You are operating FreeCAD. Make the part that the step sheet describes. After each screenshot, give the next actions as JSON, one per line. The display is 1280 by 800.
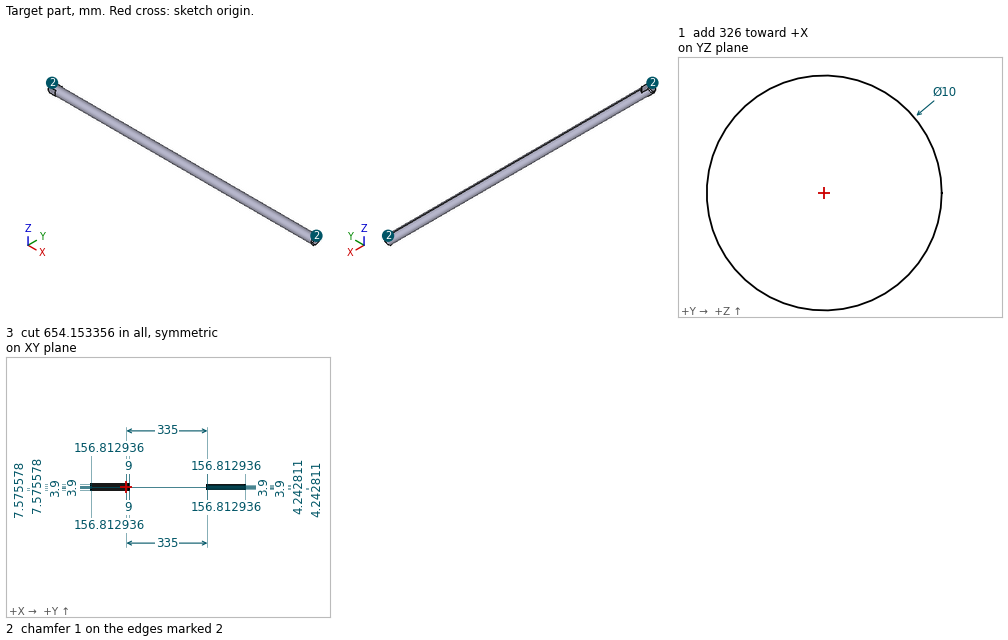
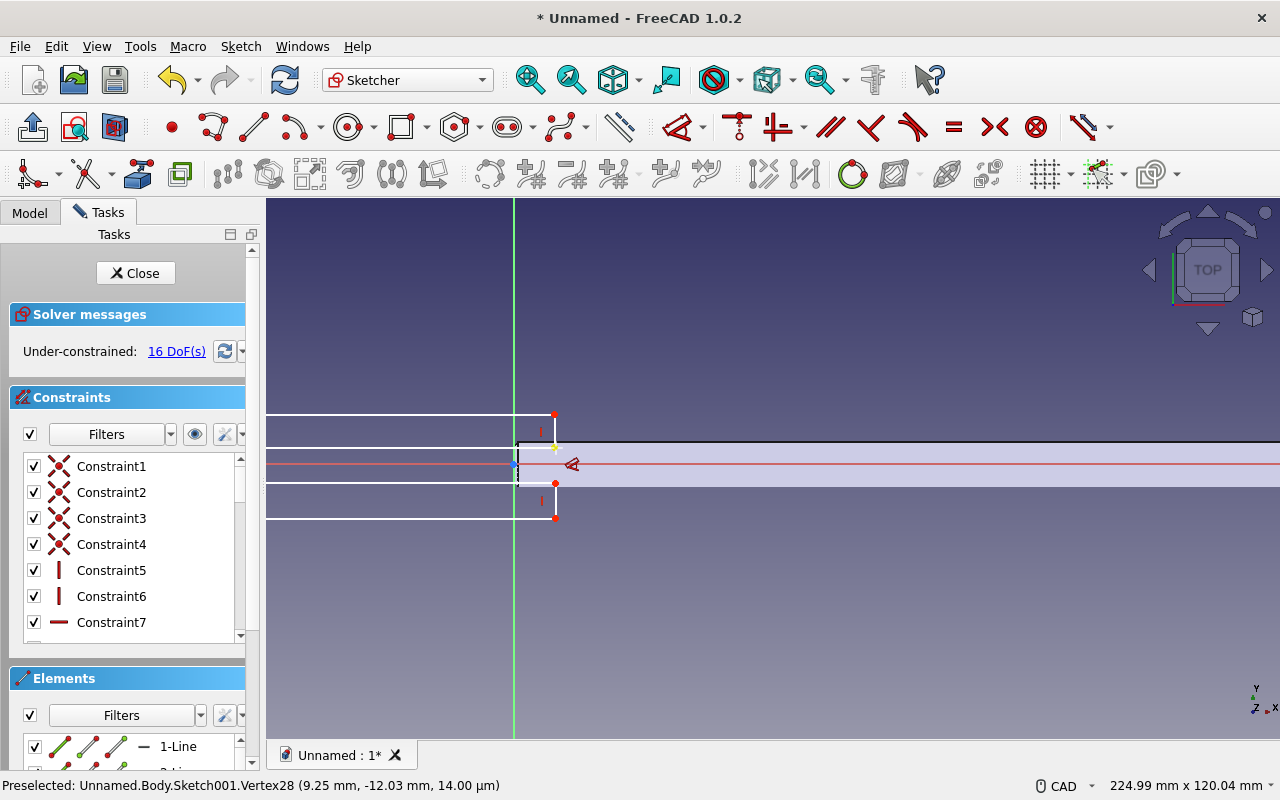
{"action": "left_click", "coordinate": [555, 448]}
{"action": "left_click", "coordinate": [534, 498]}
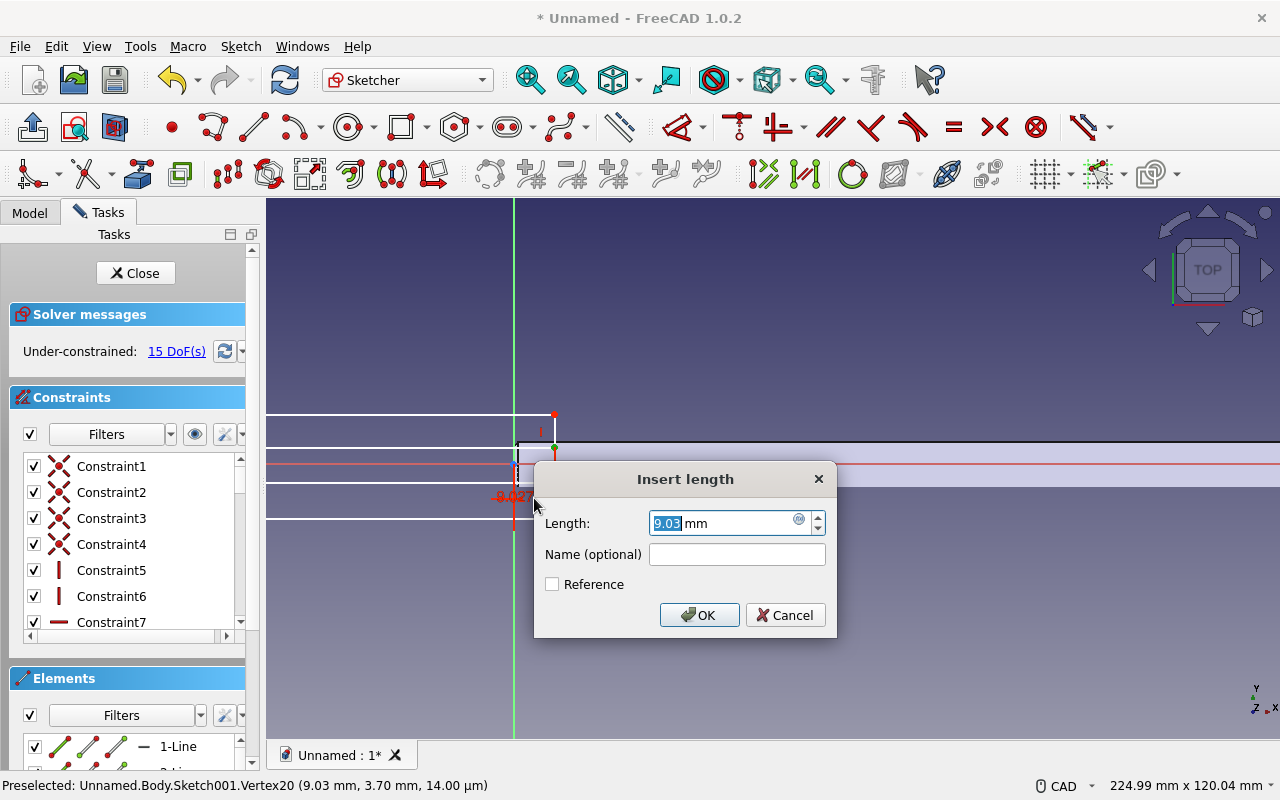
{"action": "type", "text": "9"}
{"action": "key", "text": "Return"}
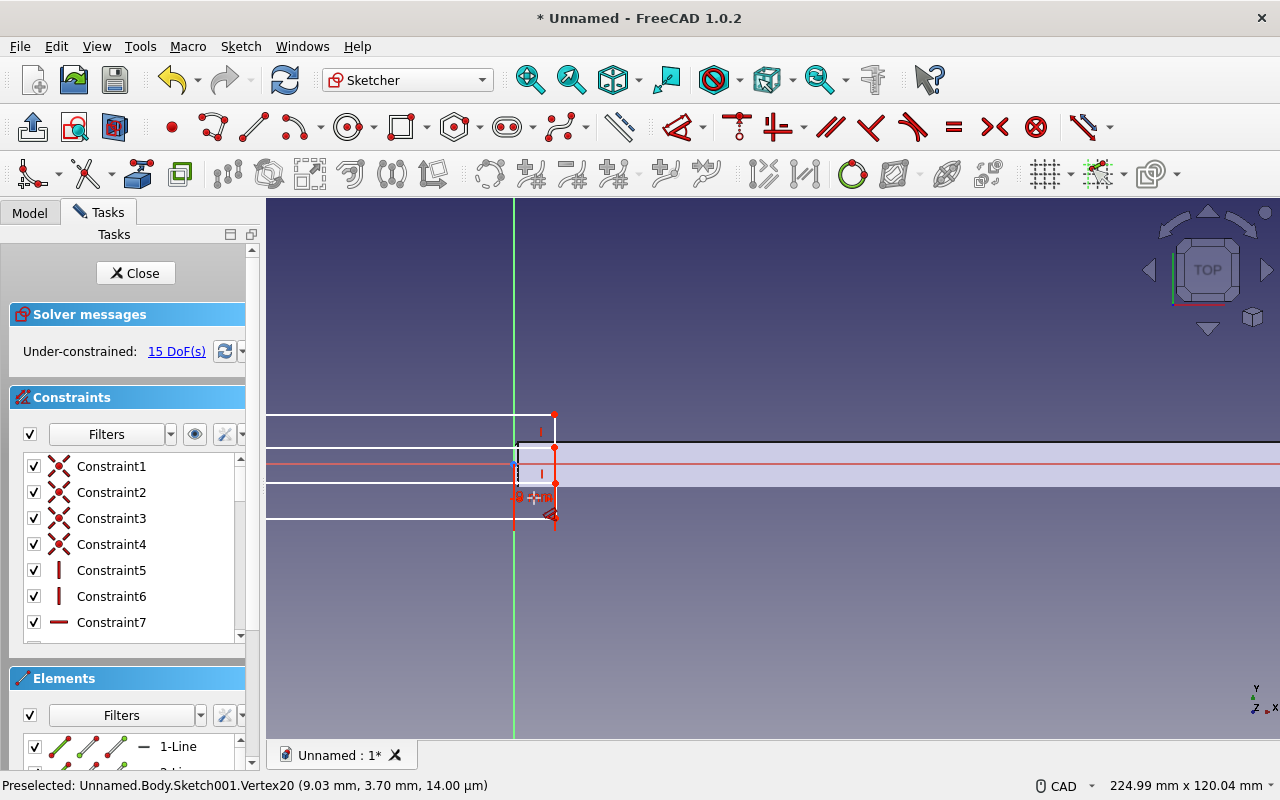
{"action": "left_click", "coordinate": [556, 519]}
{"action": "left_click", "coordinate": [535, 553]}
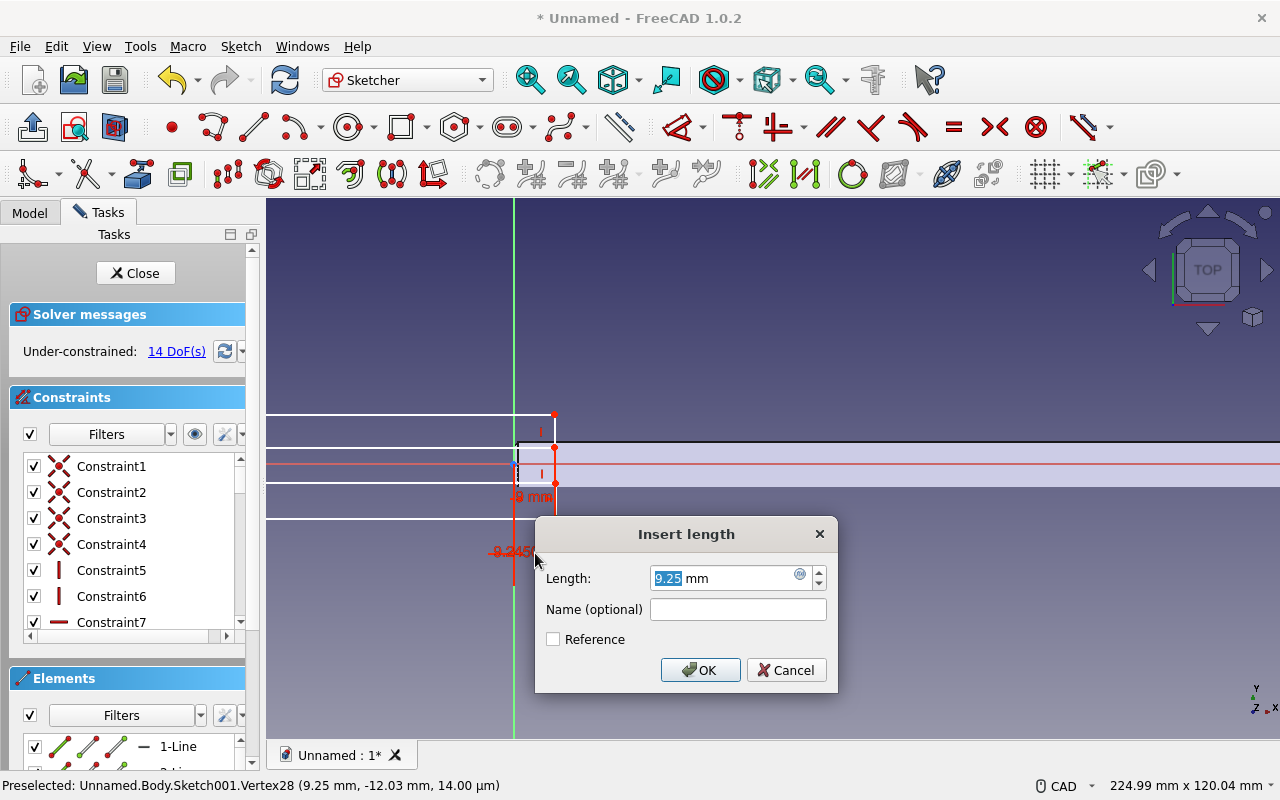
{"action": "type", "text": "9"}
{"action": "key", "text": "Return"}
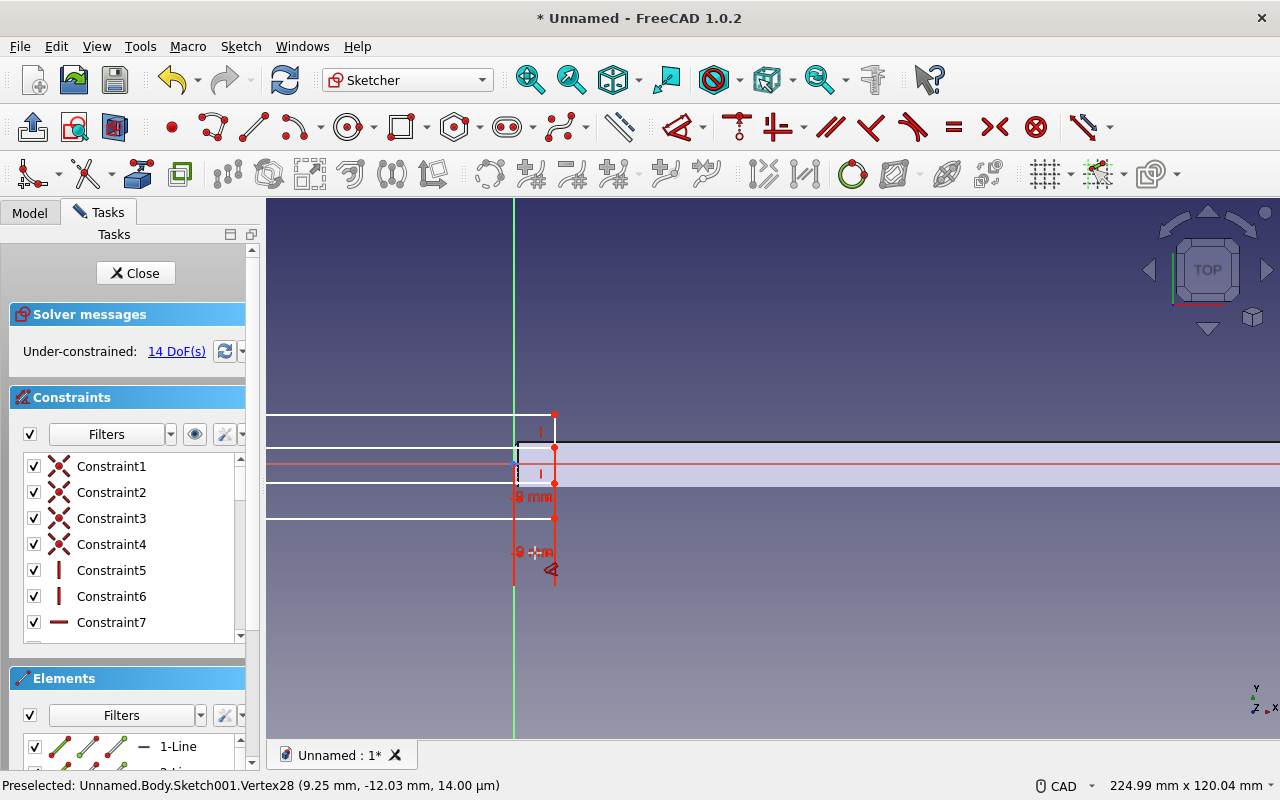
{"action": "scroll", "coordinate": [557, 470], "scroll_direction": "down", "scroll_amount": 8}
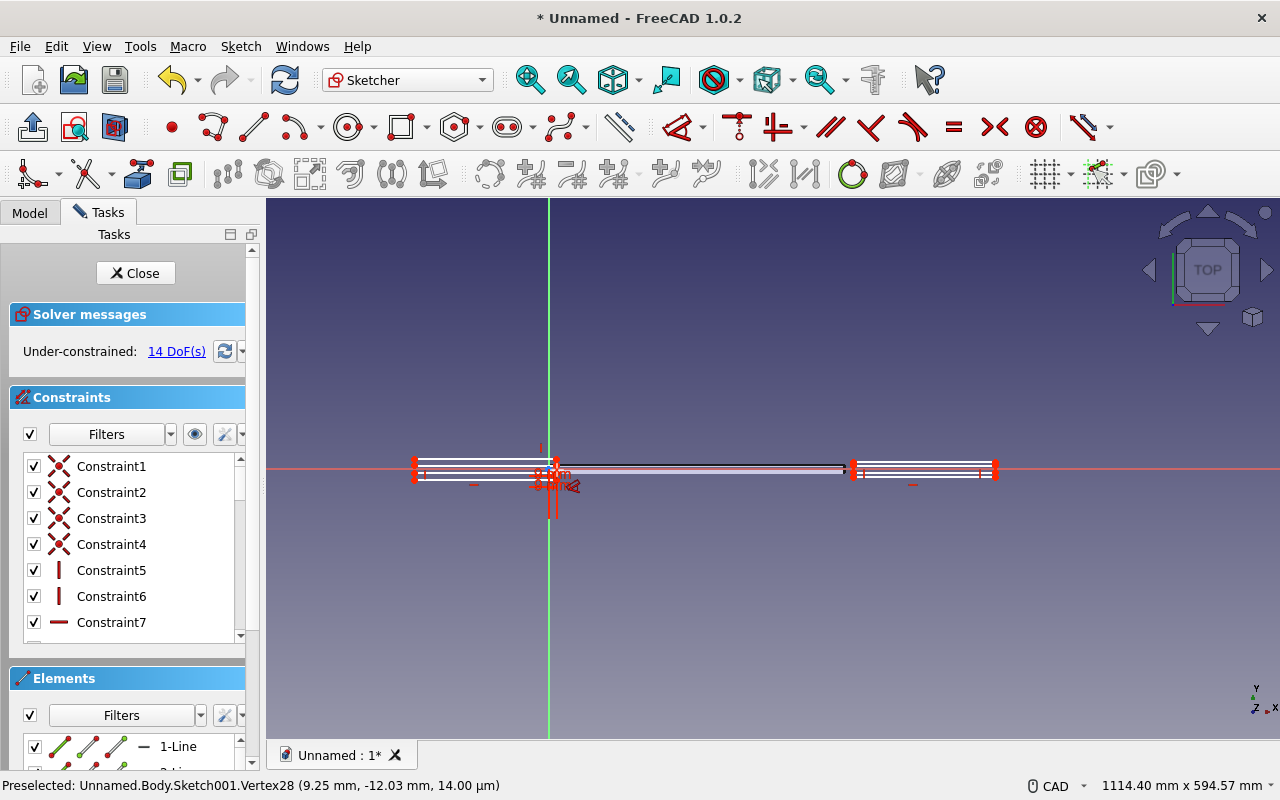
{"action": "scroll", "coordinate": [853, 462], "scroll_direction": "up", "scroll_amount": 6}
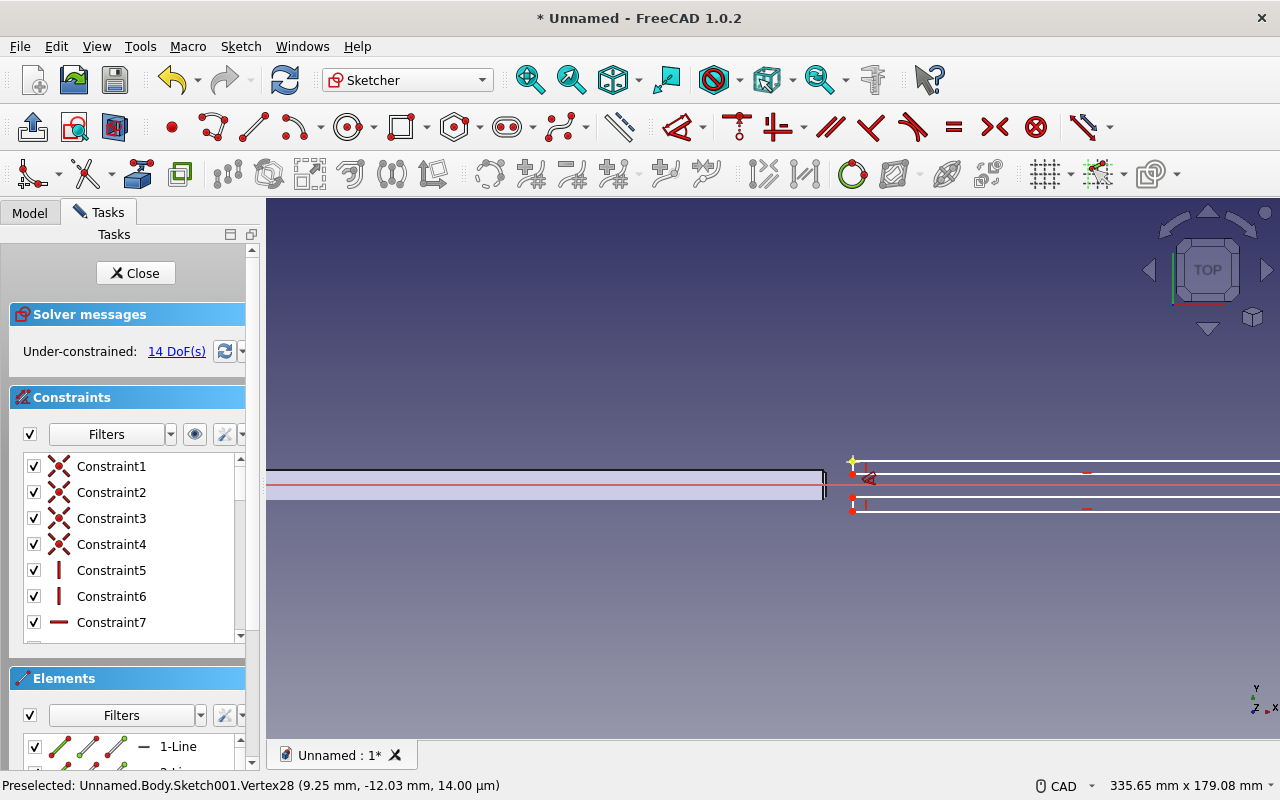
{"action": "left_click", "coordinate": [853, 461]}
{"action": "left_click", "coordinate": [573, 427]}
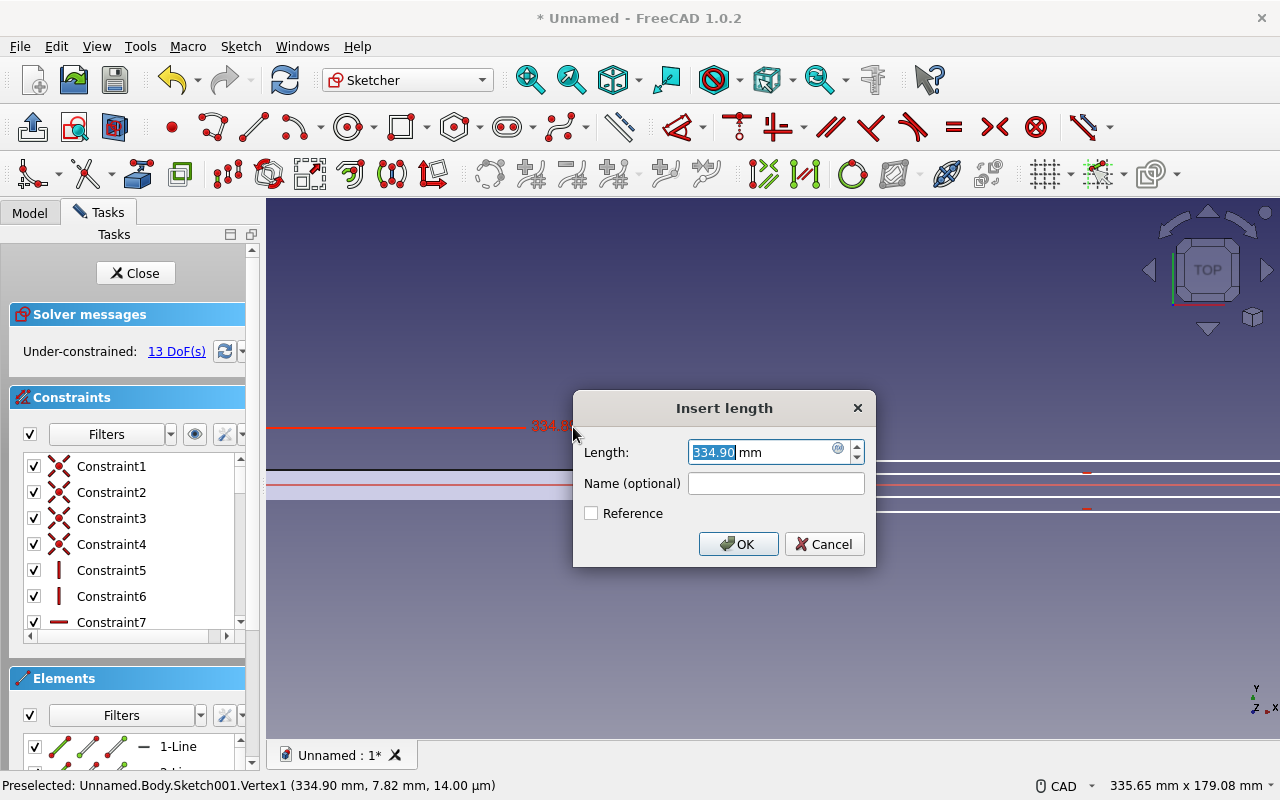
{"action": "type", "text": "335"}
{"action": "key", "text": "Return"}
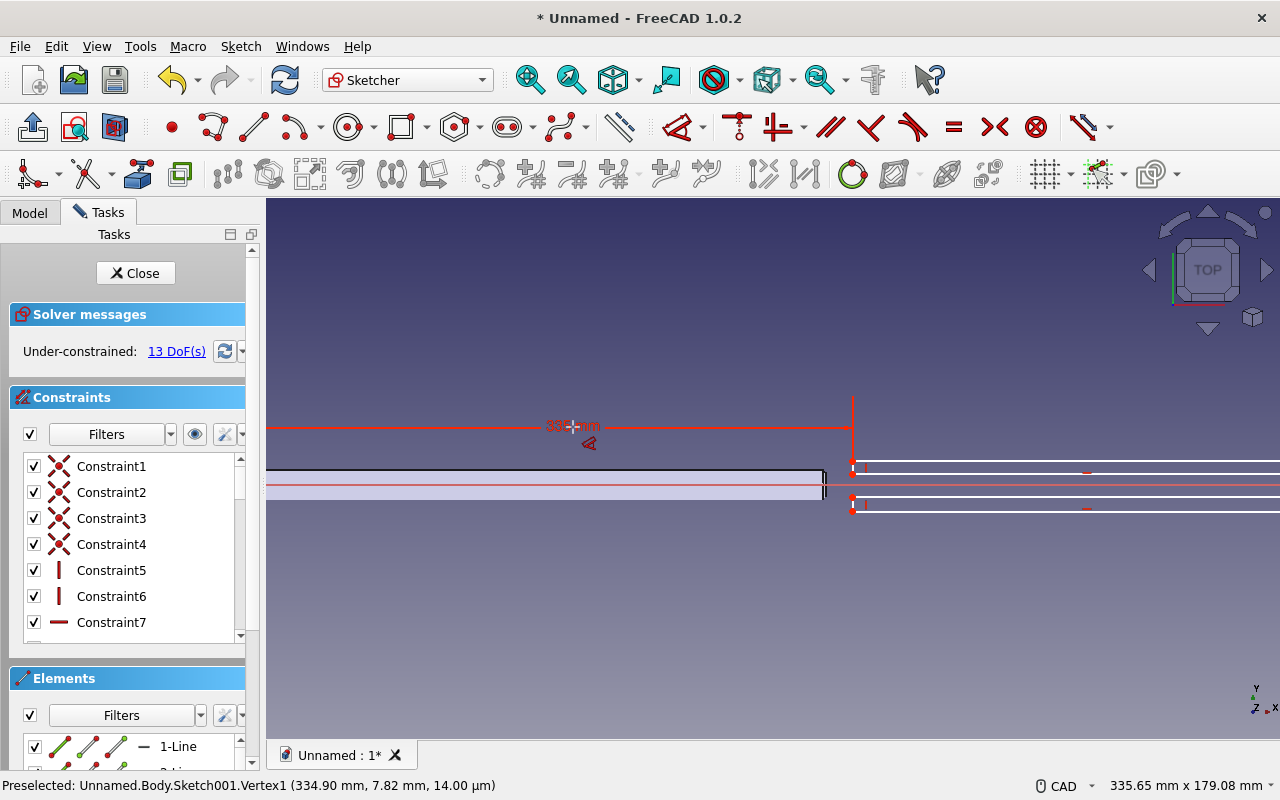
{"action": "scroll", "coordinate": [853, 474], "scroll_direction": "up", "scroll_amount": 7}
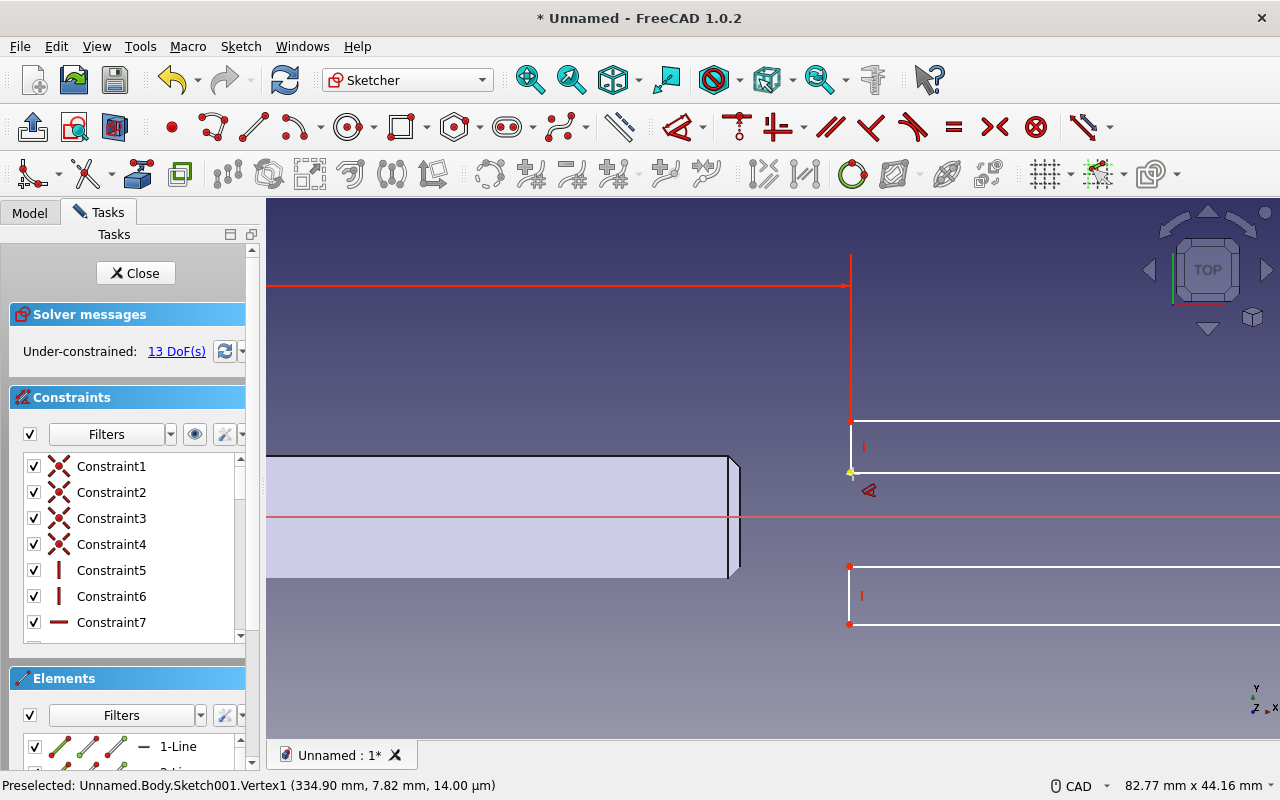
{"action": "left_click", "coordinate": [851, 473]}
{"action": "left_click", "coordinate": [885, 495]}